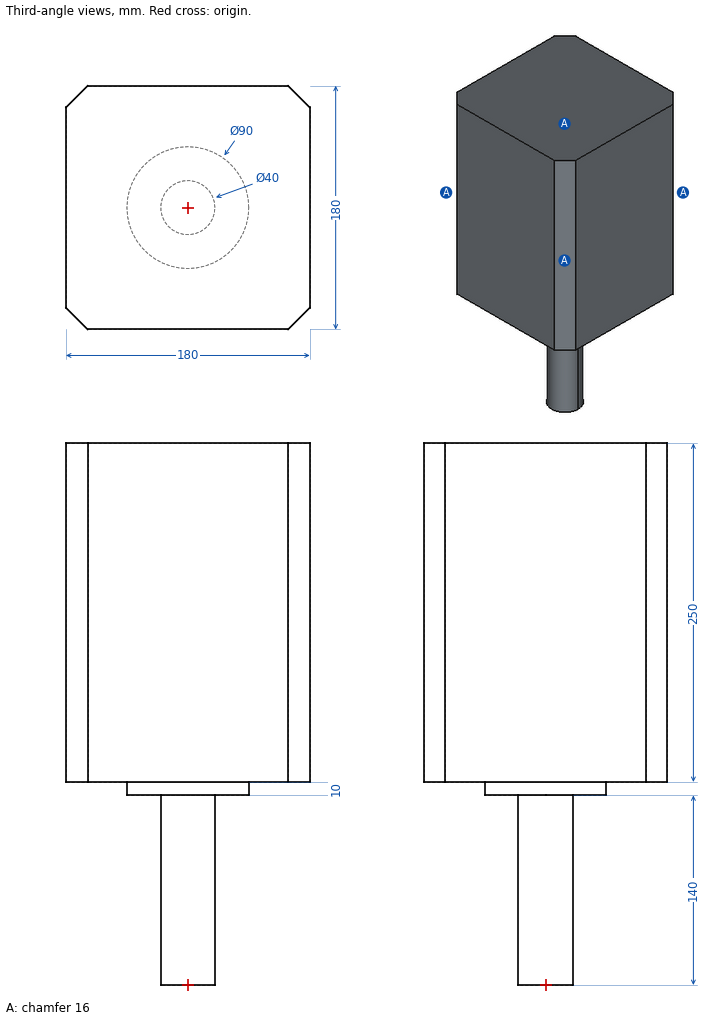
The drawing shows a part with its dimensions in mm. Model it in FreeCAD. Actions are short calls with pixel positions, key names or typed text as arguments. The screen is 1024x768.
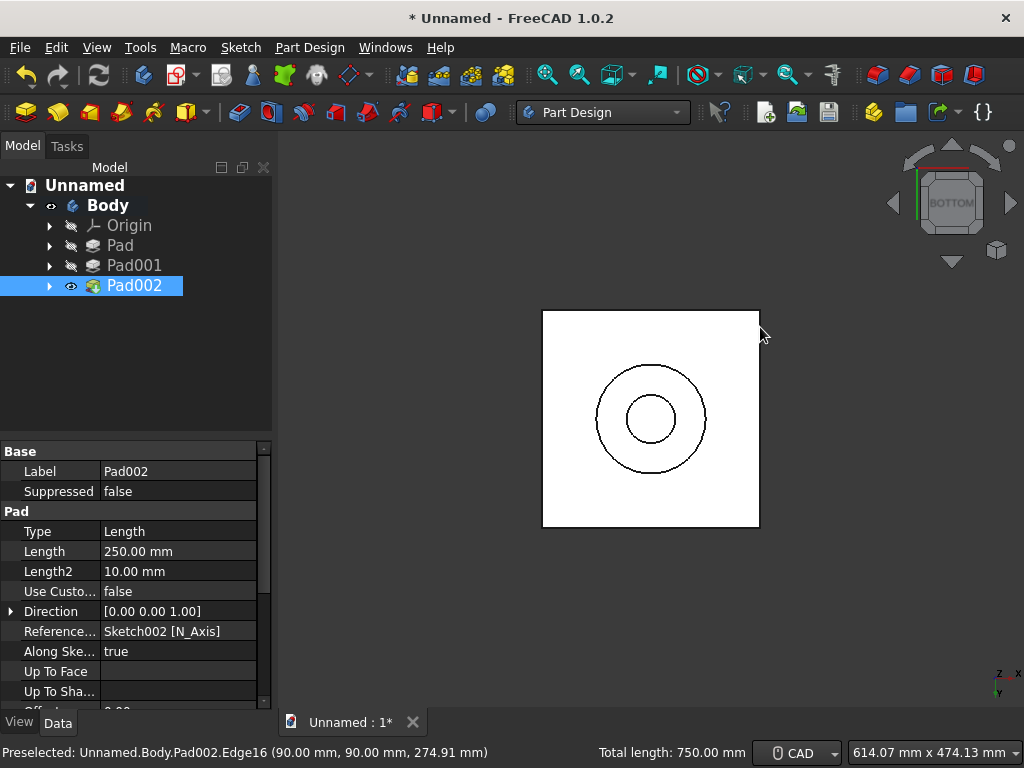
key(v)
key(f)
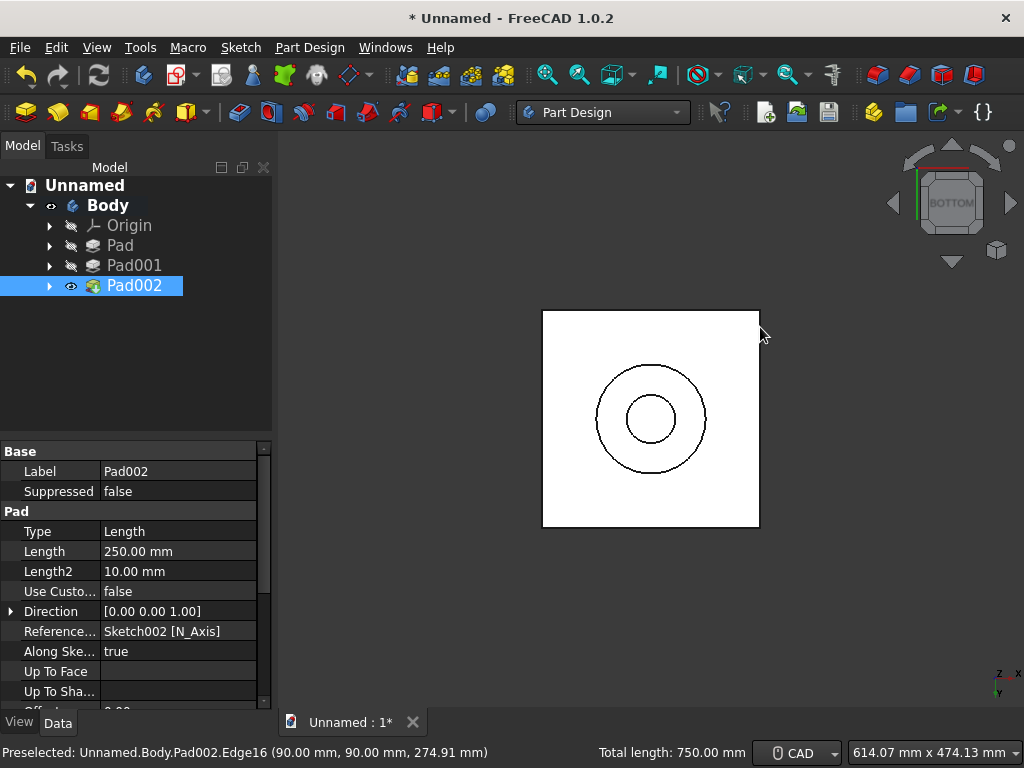
key(4)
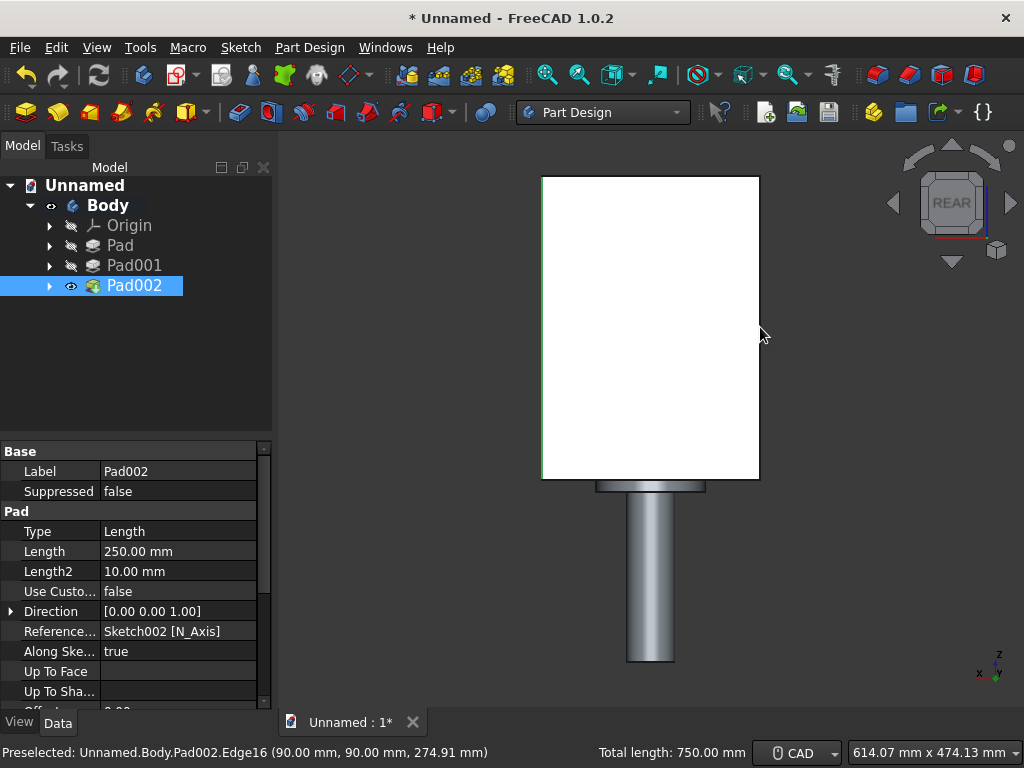
click(760, 327, ctrl)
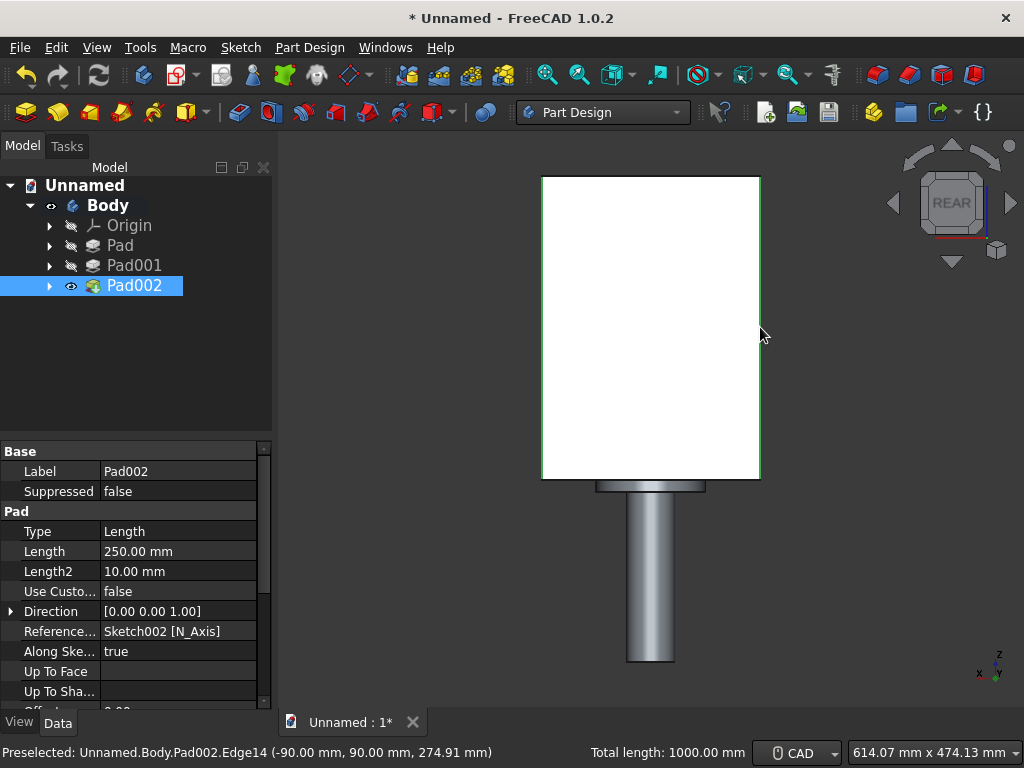
click(910, 76)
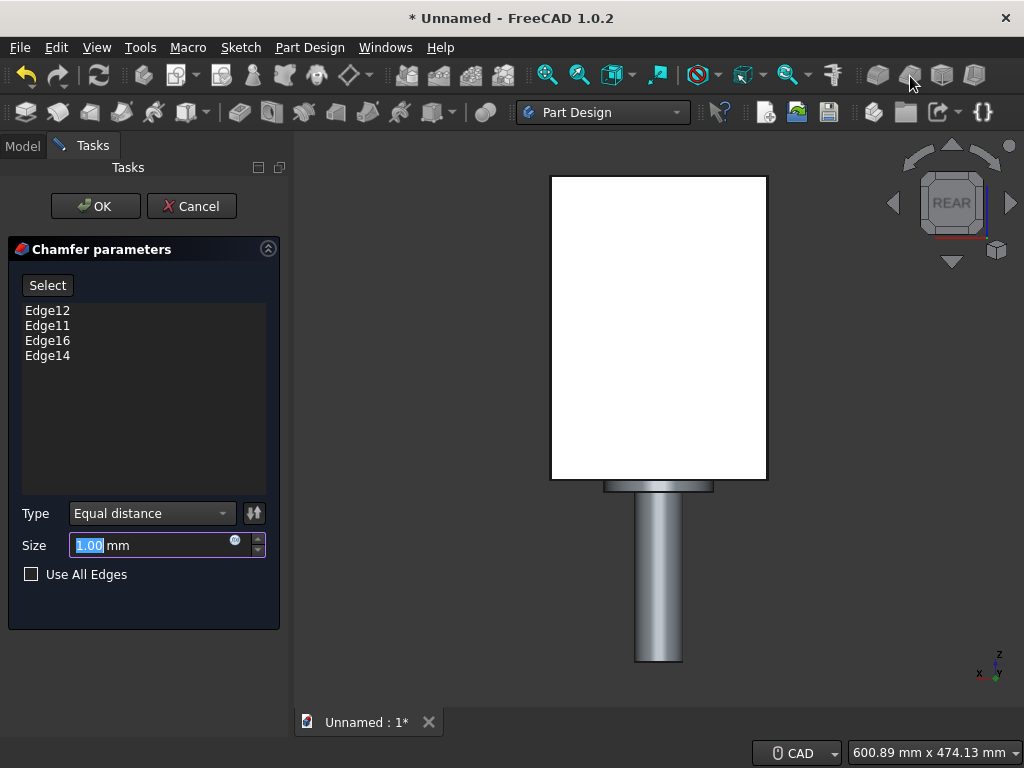
text(16)
key(Tab)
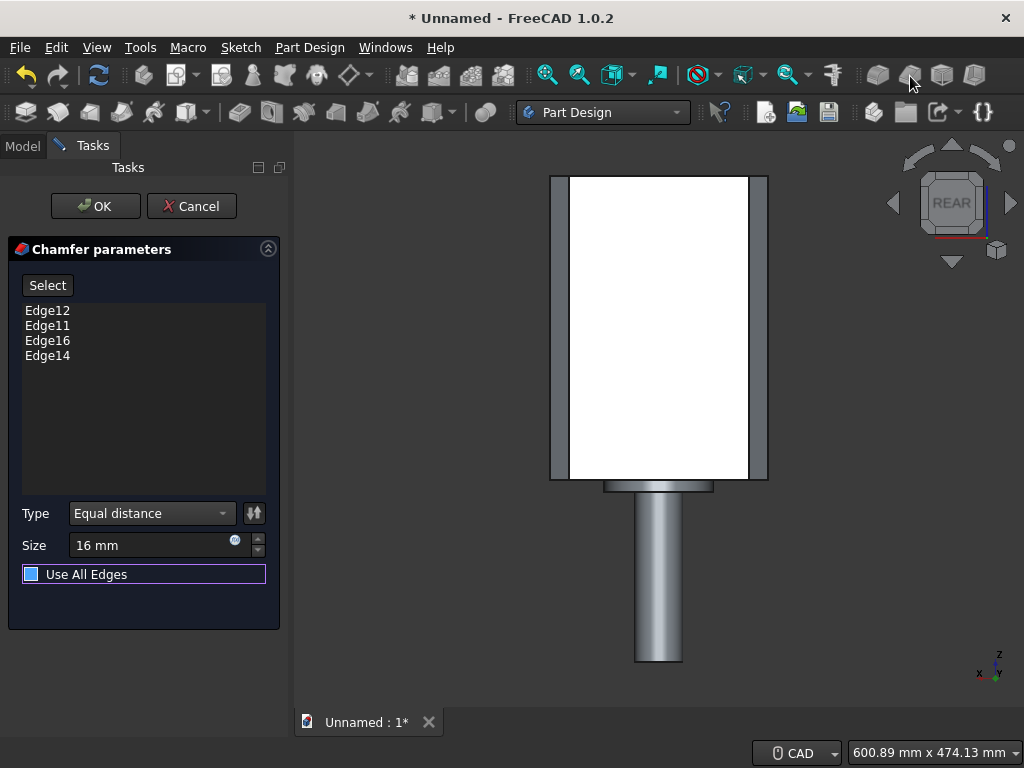
click(96, 206)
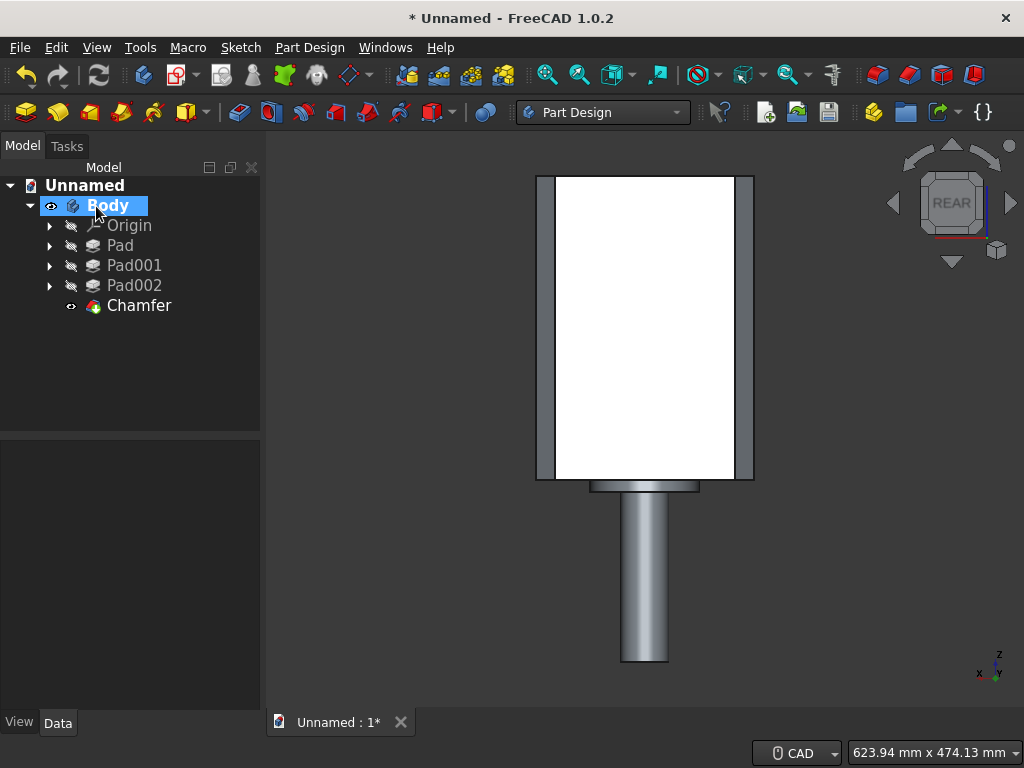
key(0)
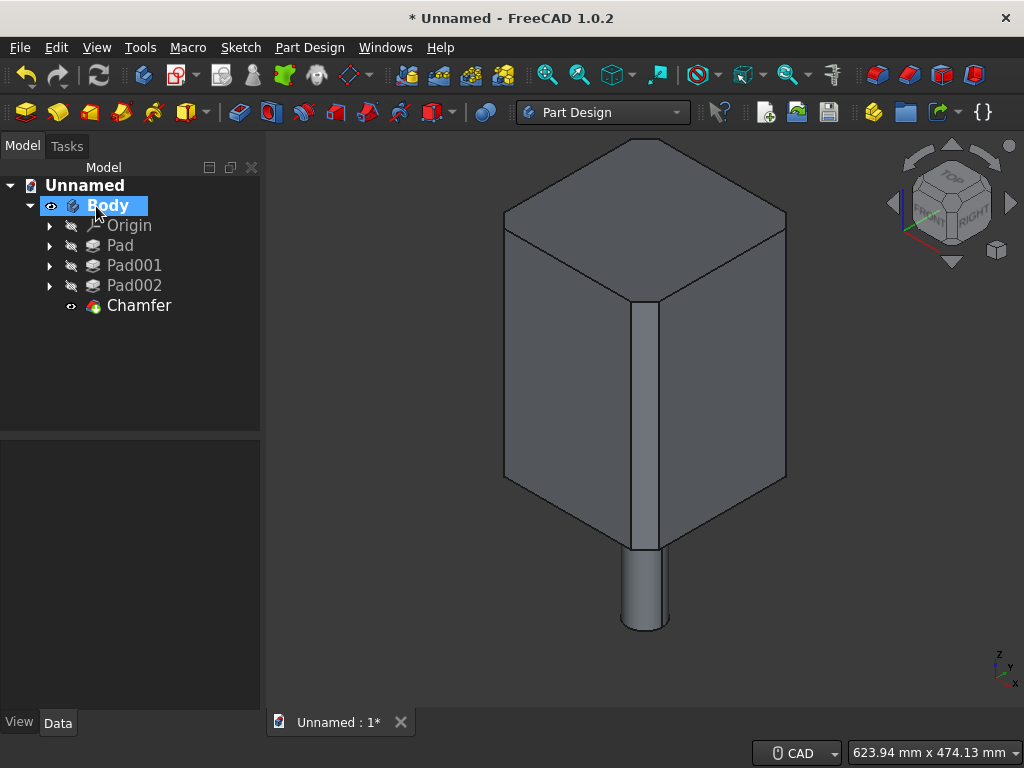
click(548, 76)